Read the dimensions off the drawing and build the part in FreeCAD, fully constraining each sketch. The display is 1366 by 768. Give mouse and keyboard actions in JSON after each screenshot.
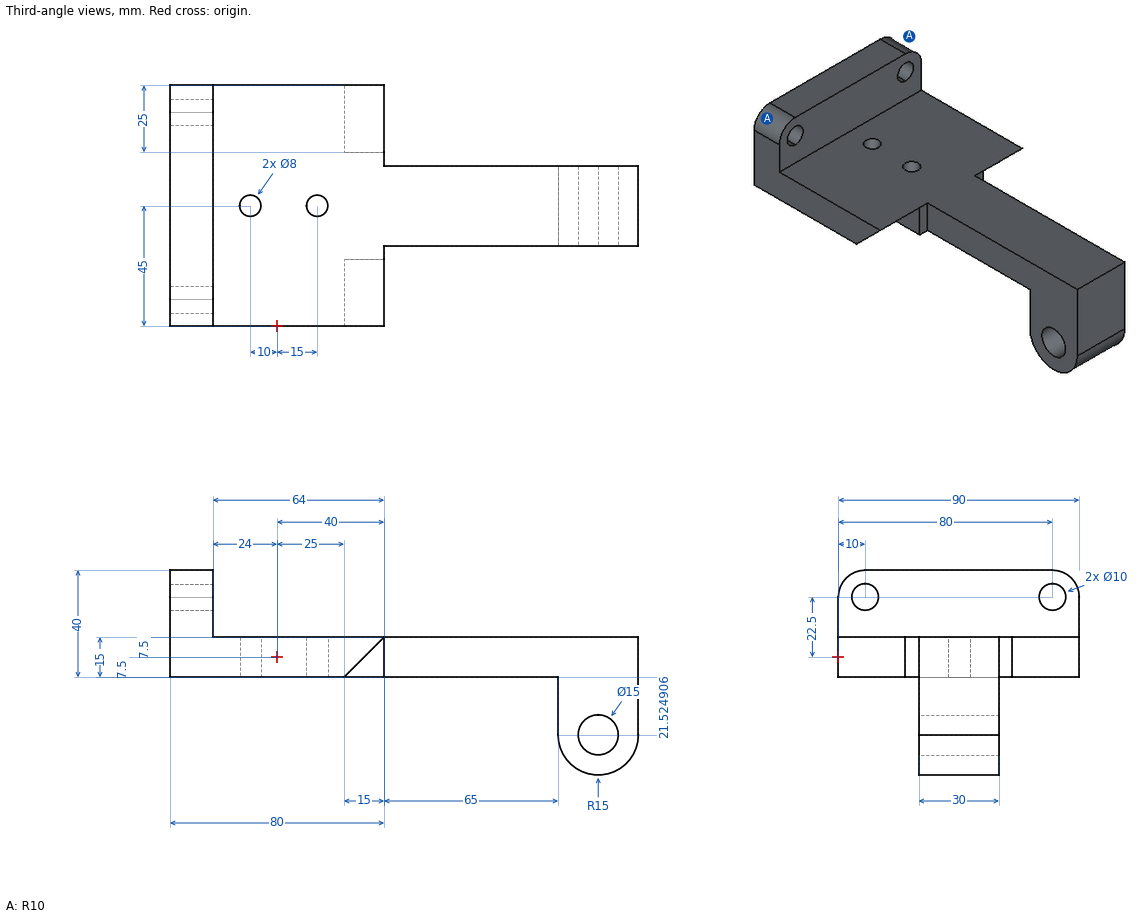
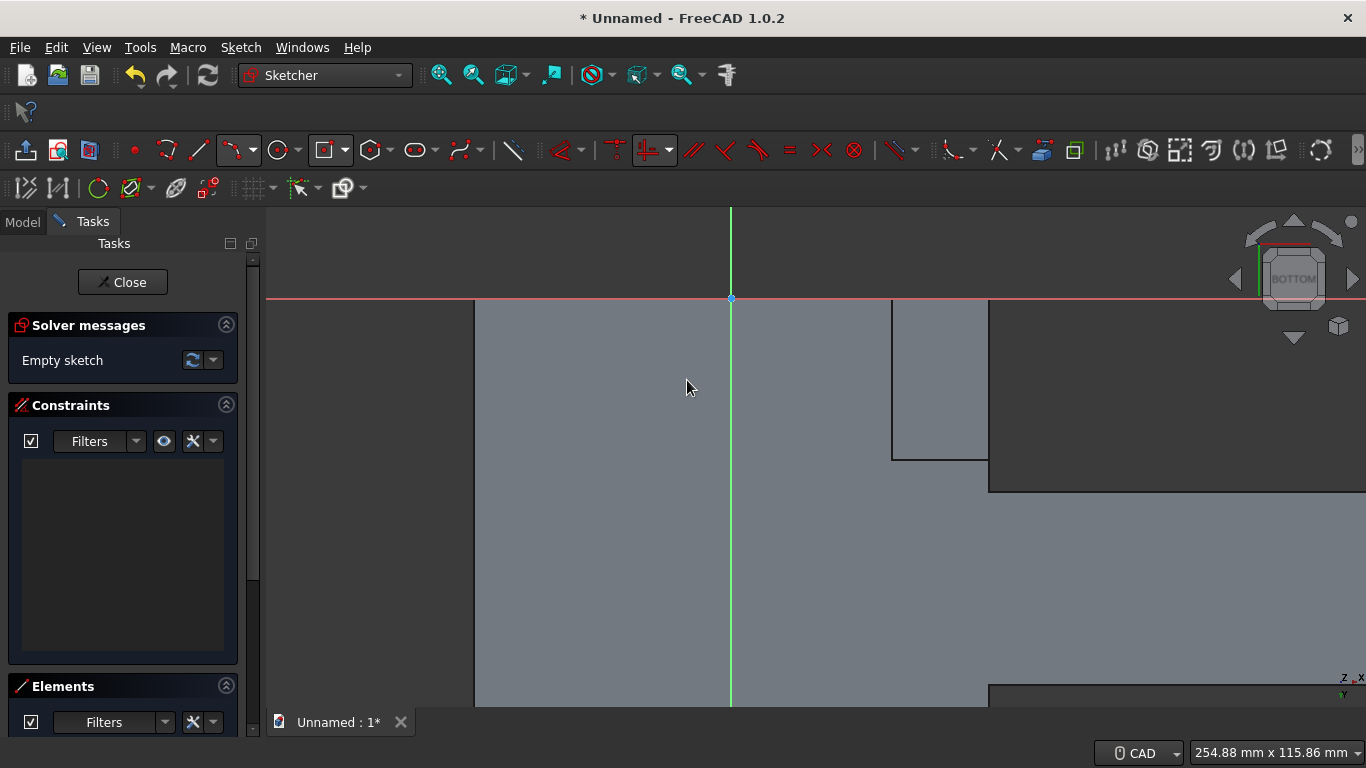
{"action": "left_click", "coordinate": [278, 150]}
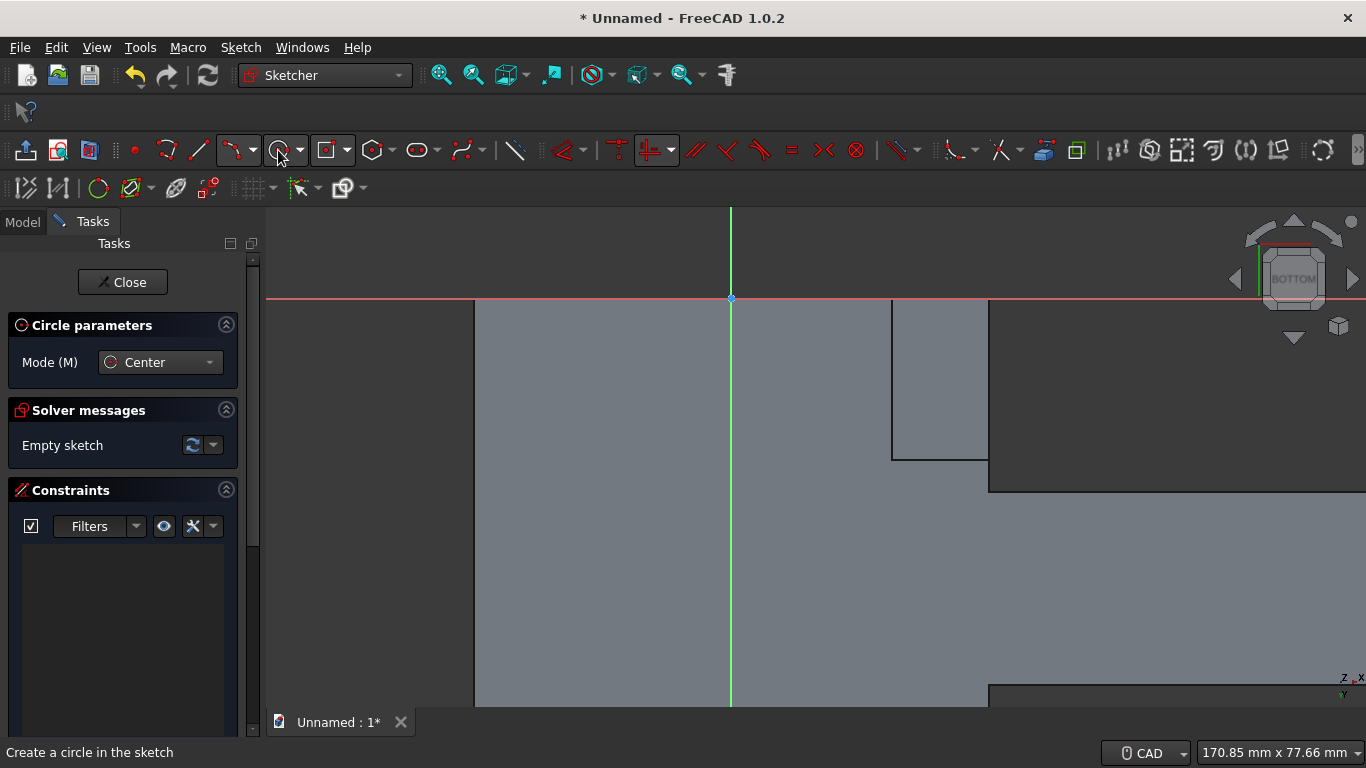
{"action": "left_click", "coordinate": [667, 589]}
{"action": "left_click", "coordinate": [685, 571]}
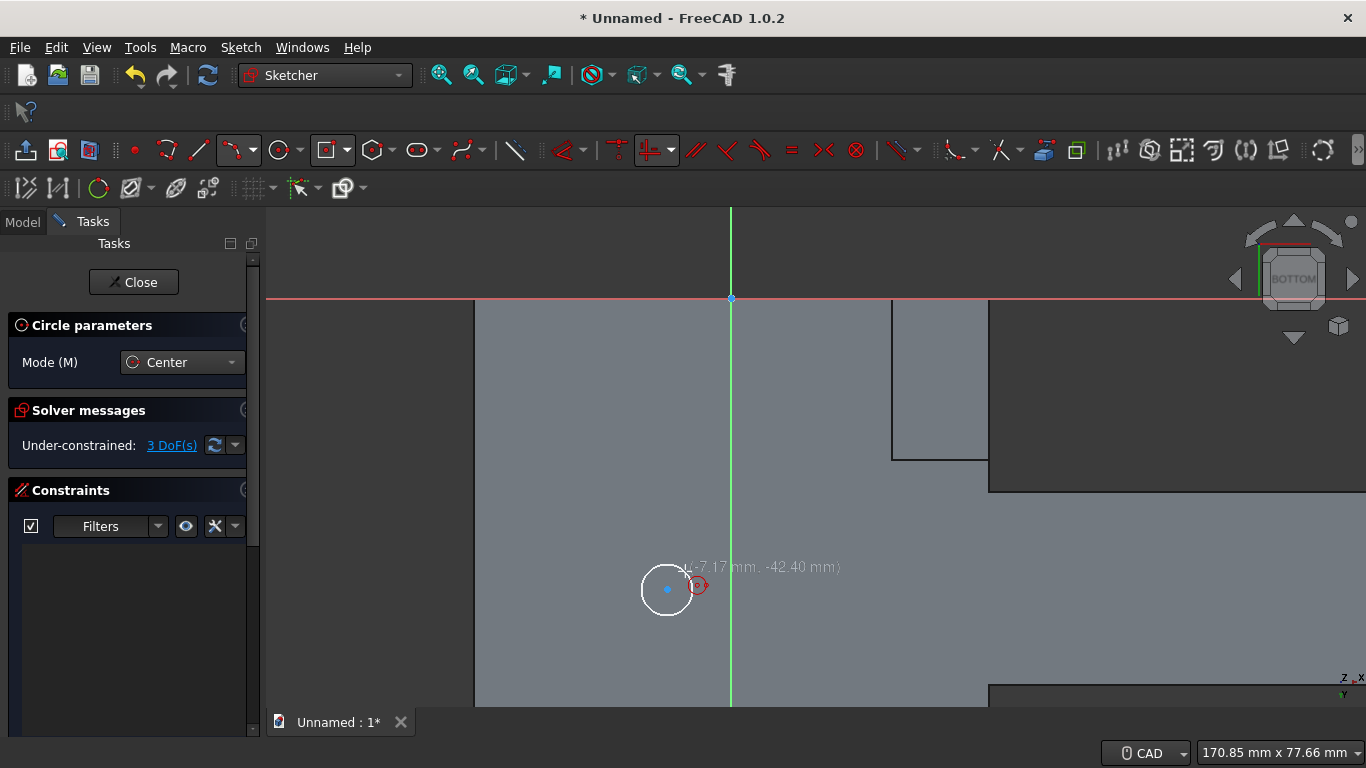
{"action": "left_click", "coordinate": [828, 589]}
{"action": "left_click", "coordinate": [846, 571]}
{"action": "key", "text": "Escape"}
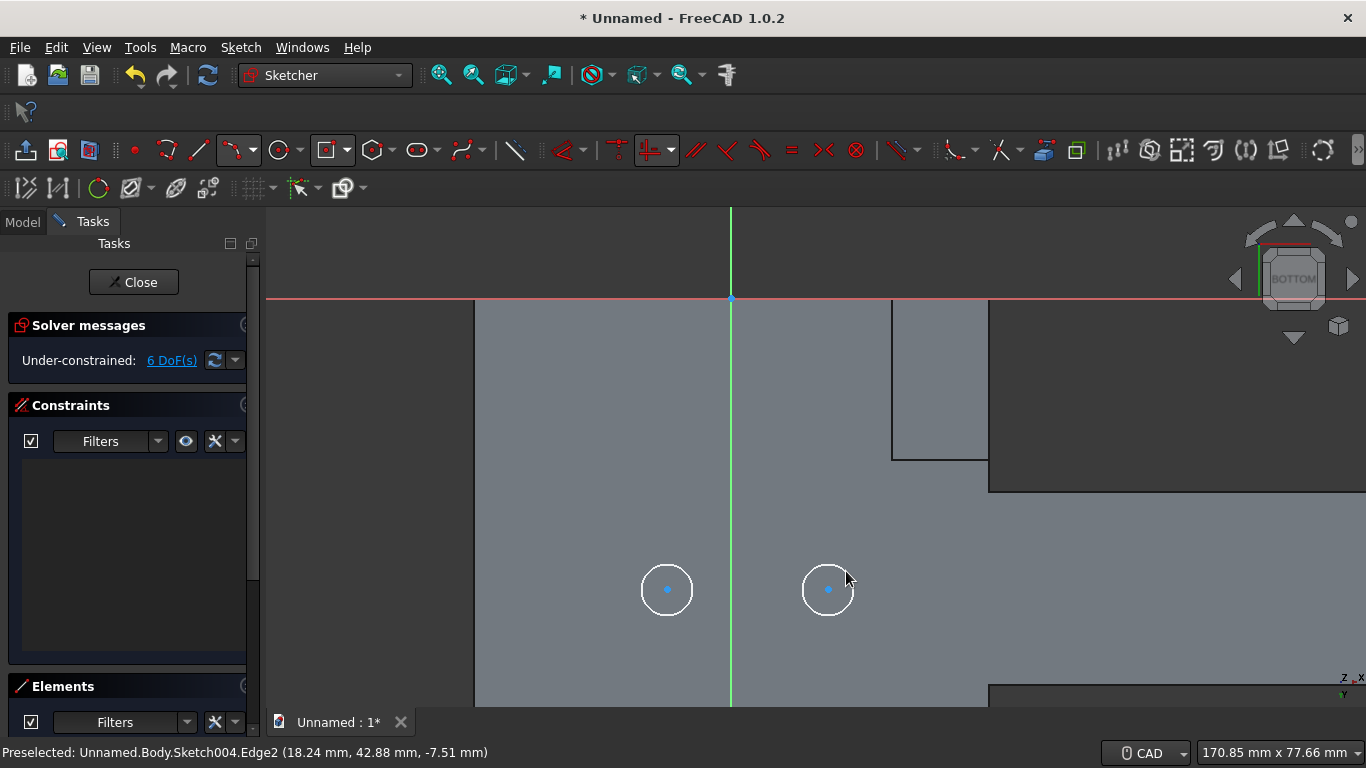
{"action": "left_click", "coordinate": [685, 572]}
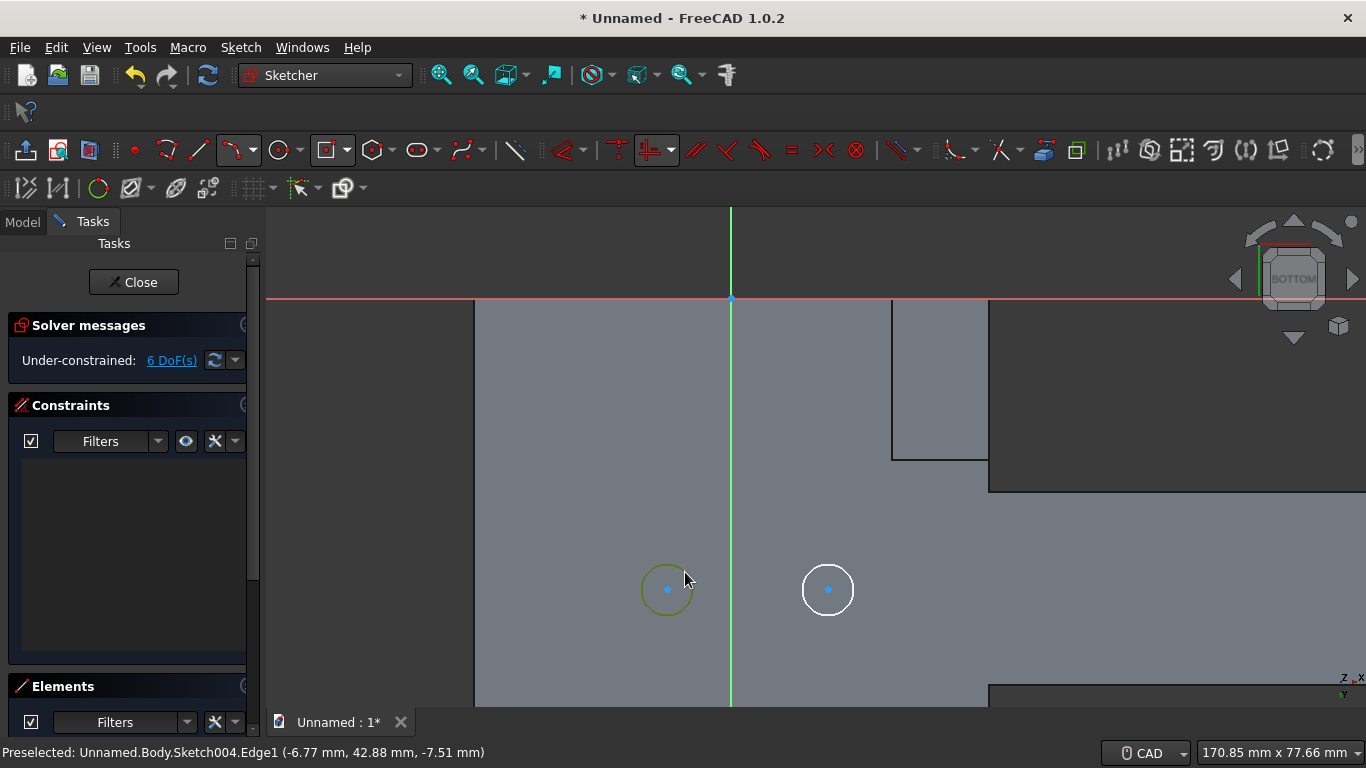
{"action": "left_click", "coordinate": [846, 572]}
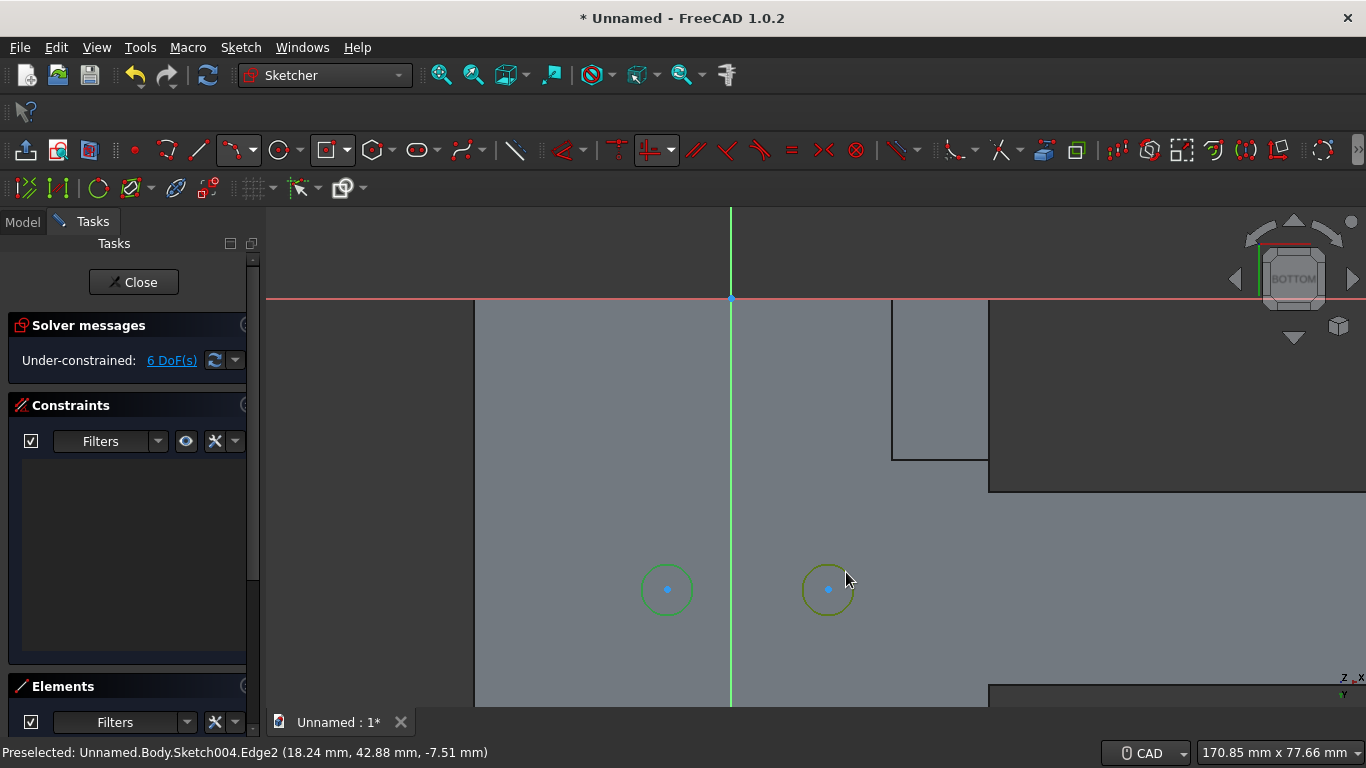
{"action": "left_click", "coordinate": [792, 150]}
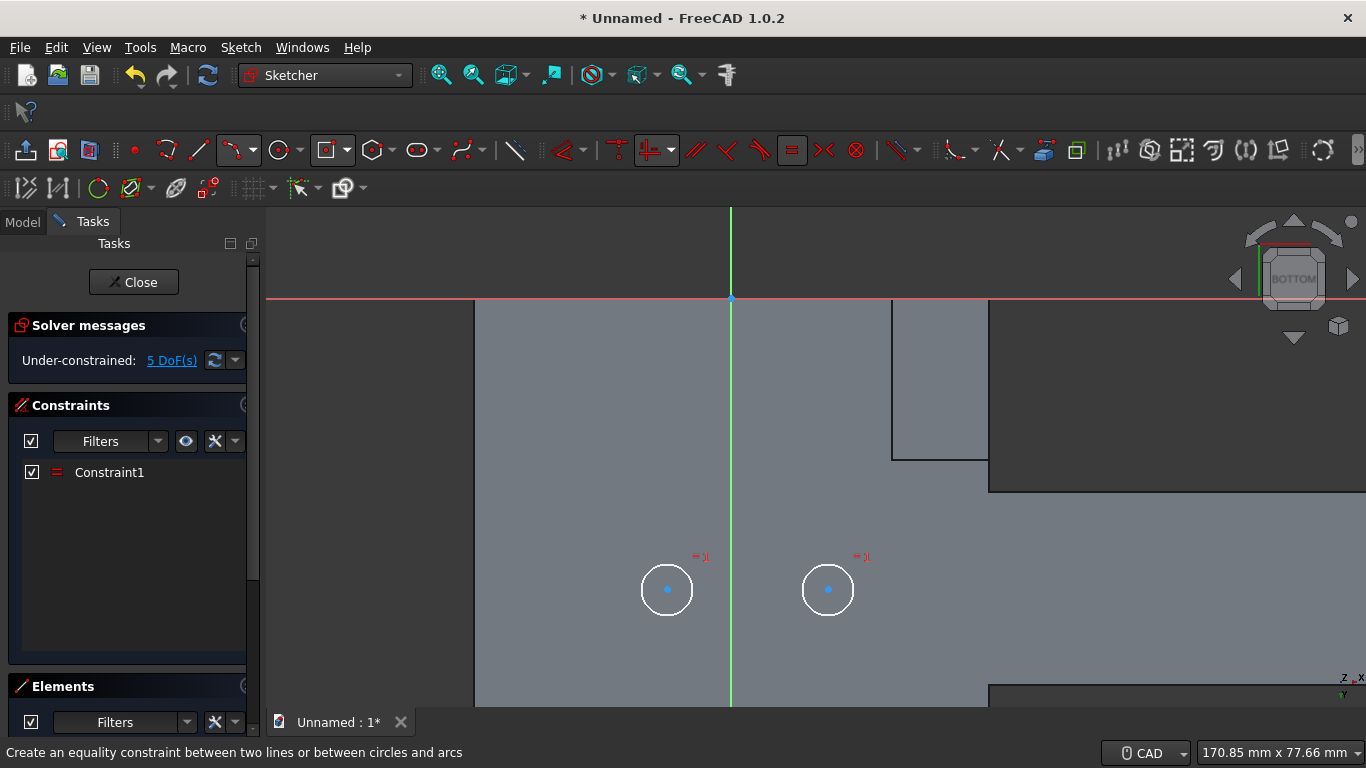
{"action": "left_click", "coordinate": [667, 590]}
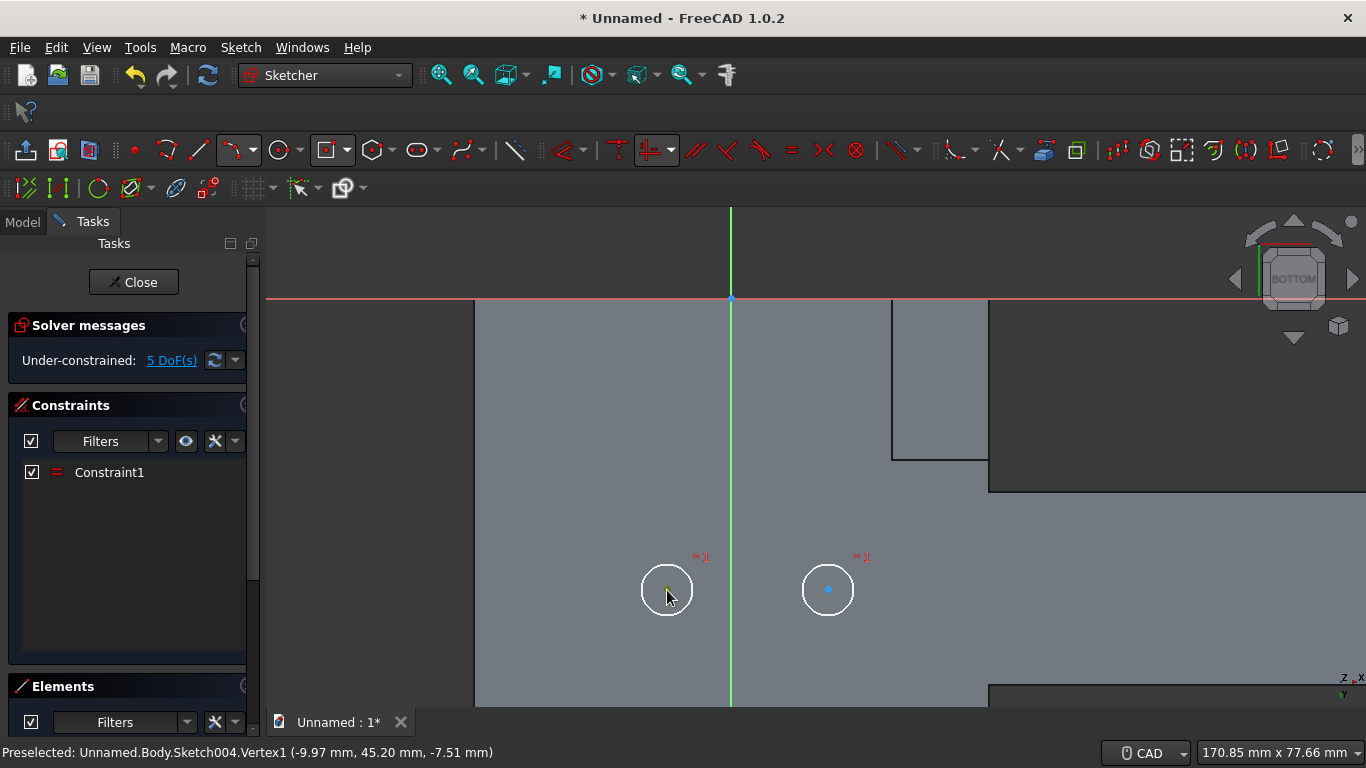
{"action": "left_click", "coordinate": [828, 590]}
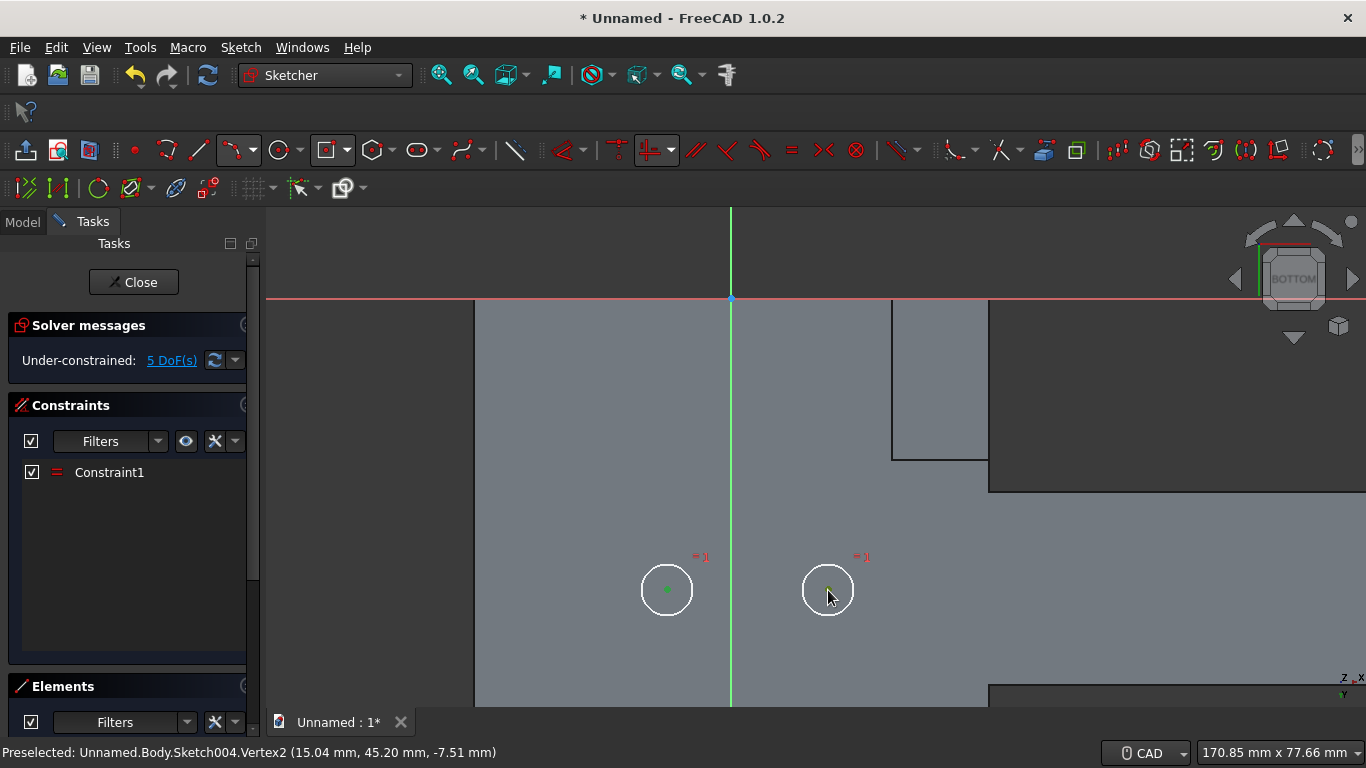
{"action": "key", "text": "h"}